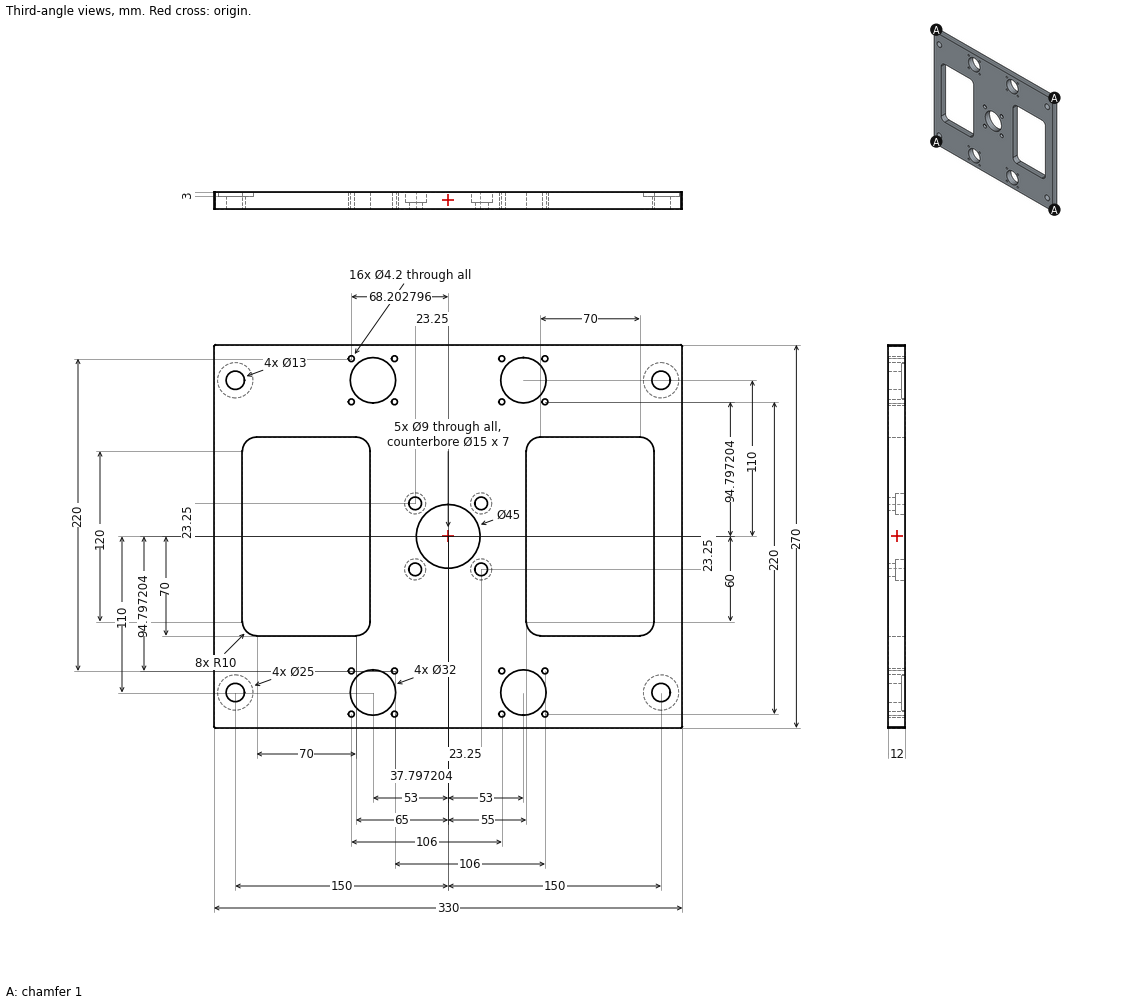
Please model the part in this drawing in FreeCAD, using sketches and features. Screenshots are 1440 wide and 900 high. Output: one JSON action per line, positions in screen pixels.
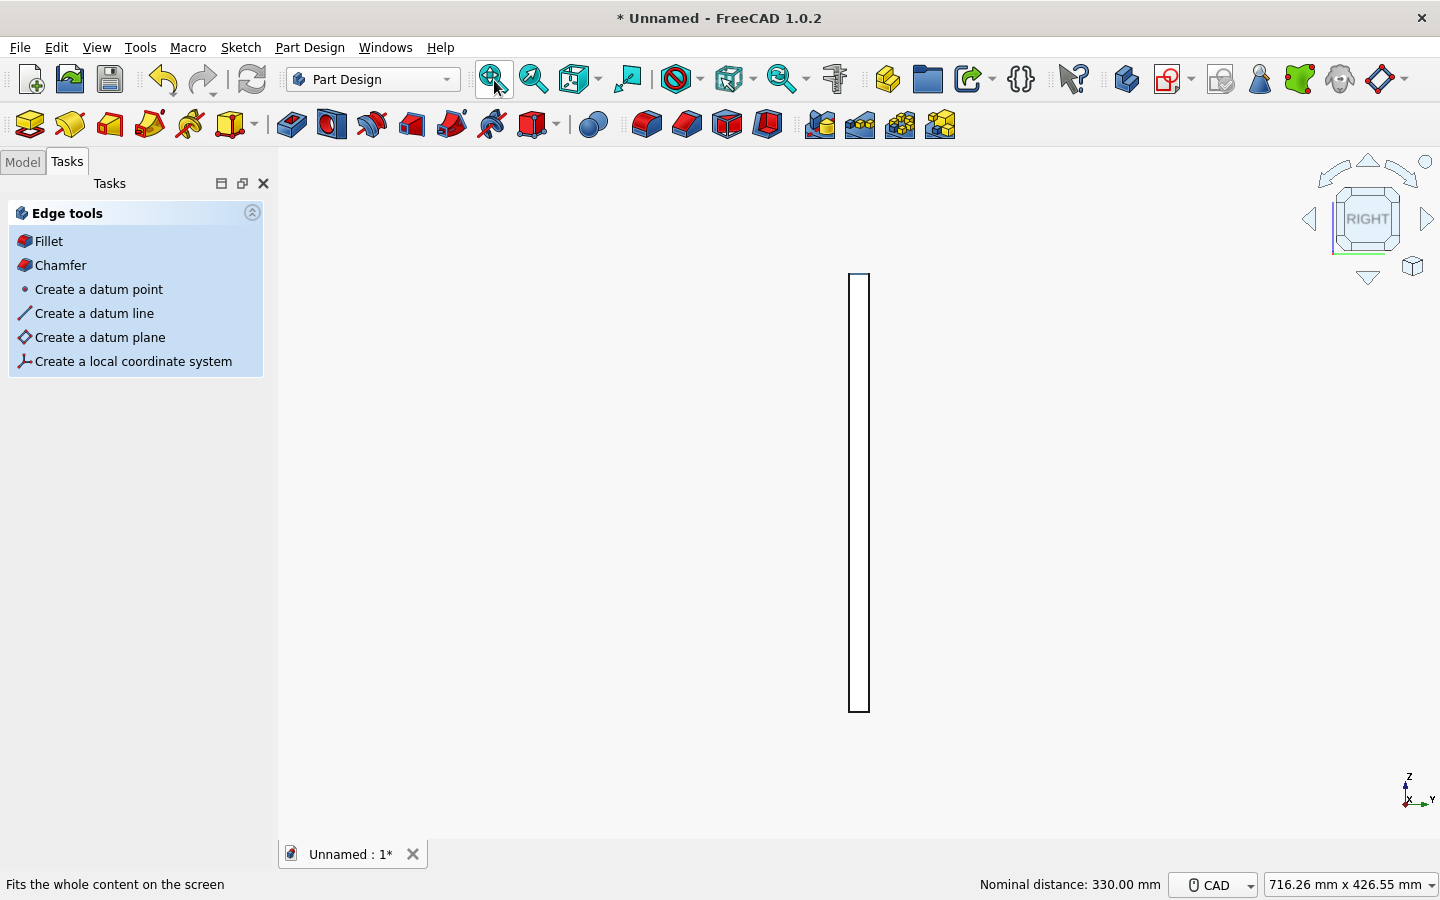
{"action": "left_click", "coordinate": [859, 711], "text": "ctrl"}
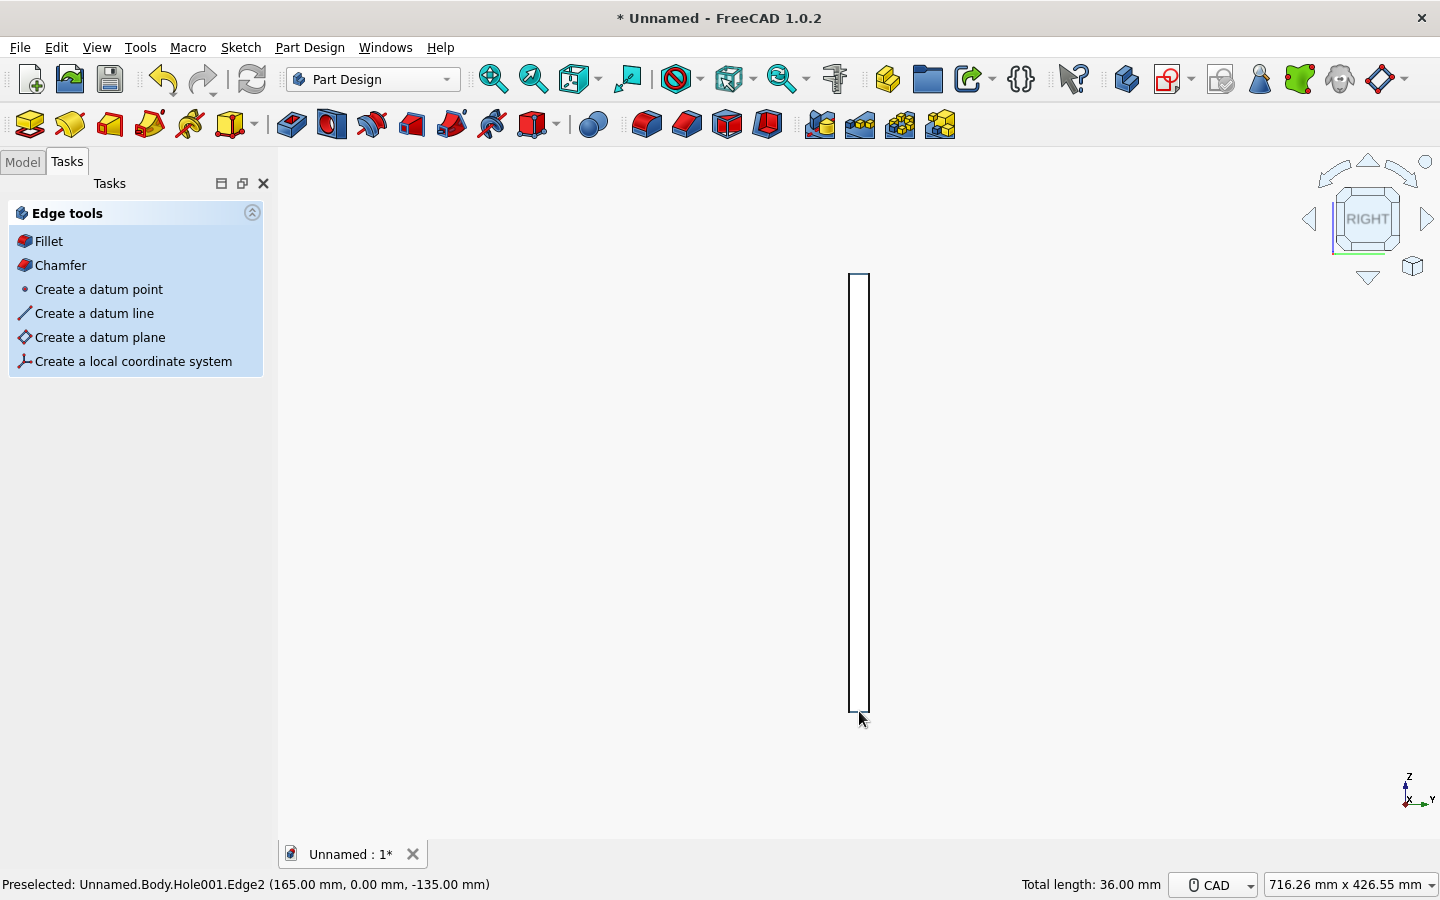
{"action": "scroll", "coordinate": [859, 711], "scroll_direction": "up", "scroll_amount": 4}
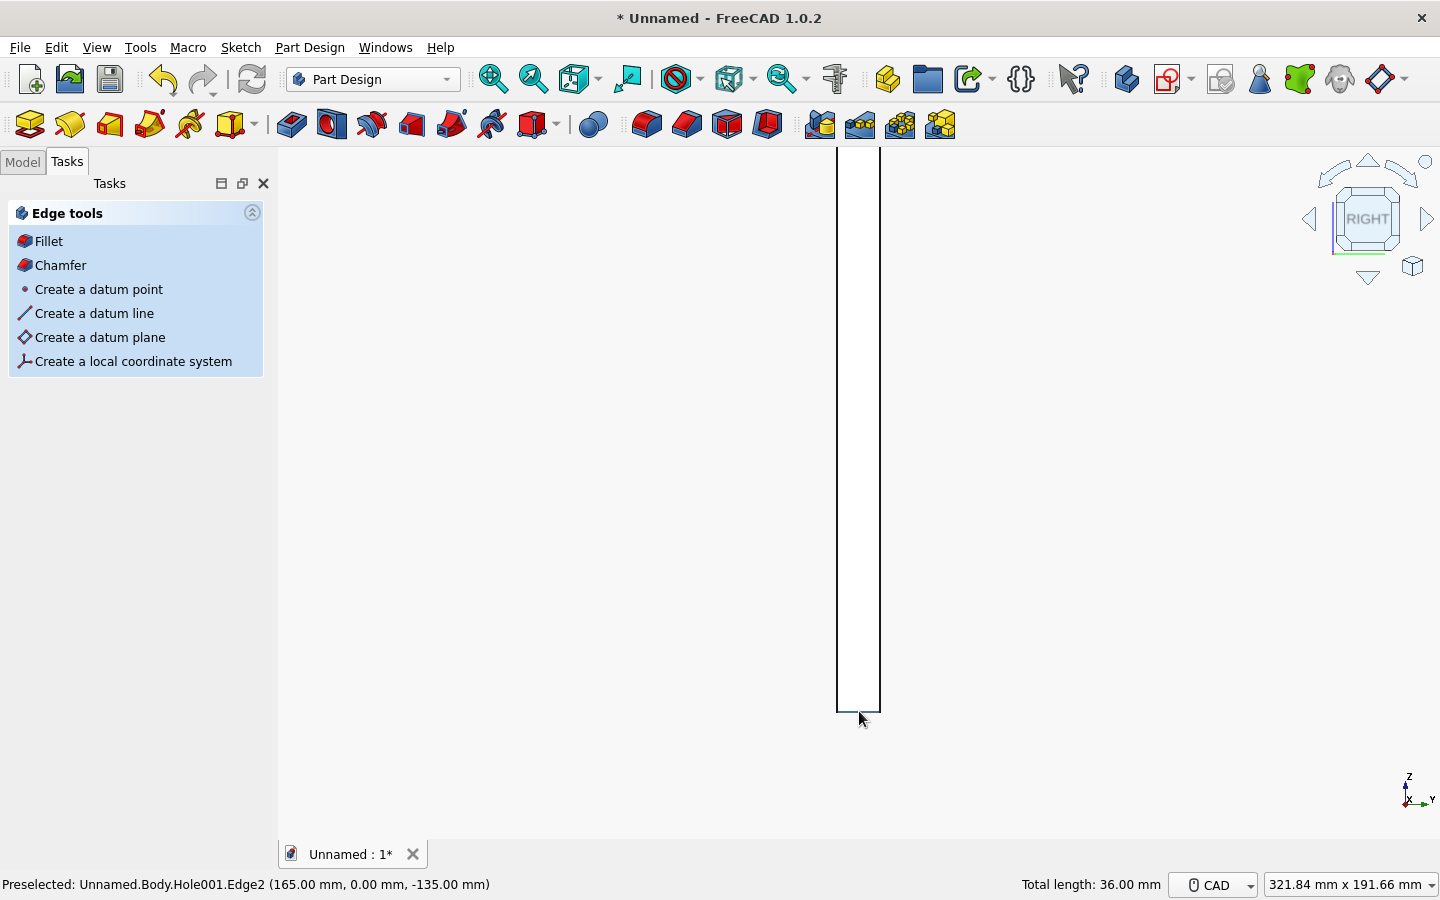
{"action": "left_click", "coordinate": [494, 80]}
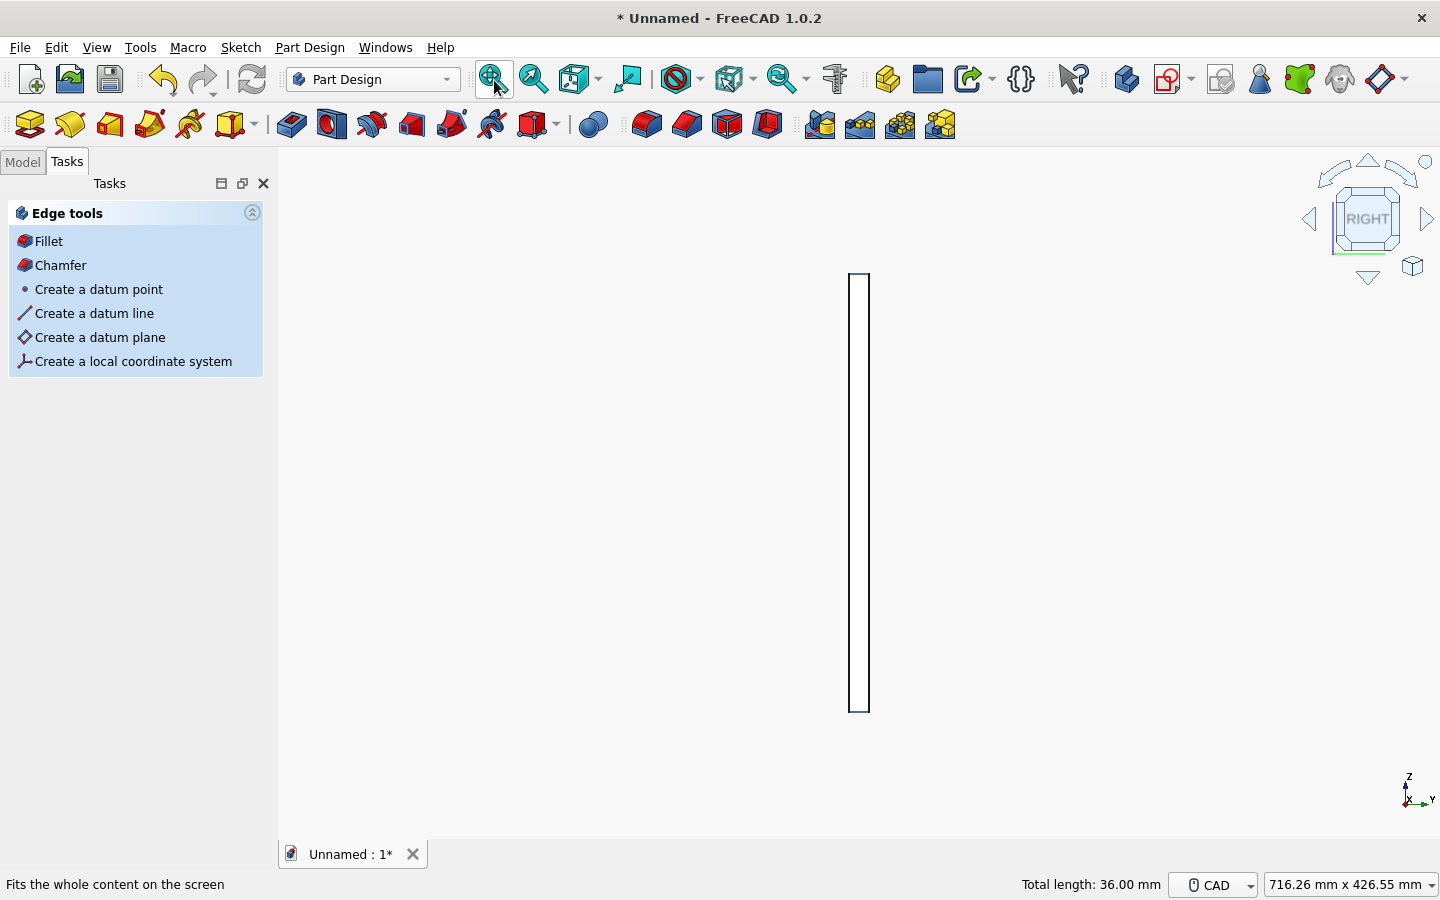
{"action": "key", "text": "5"}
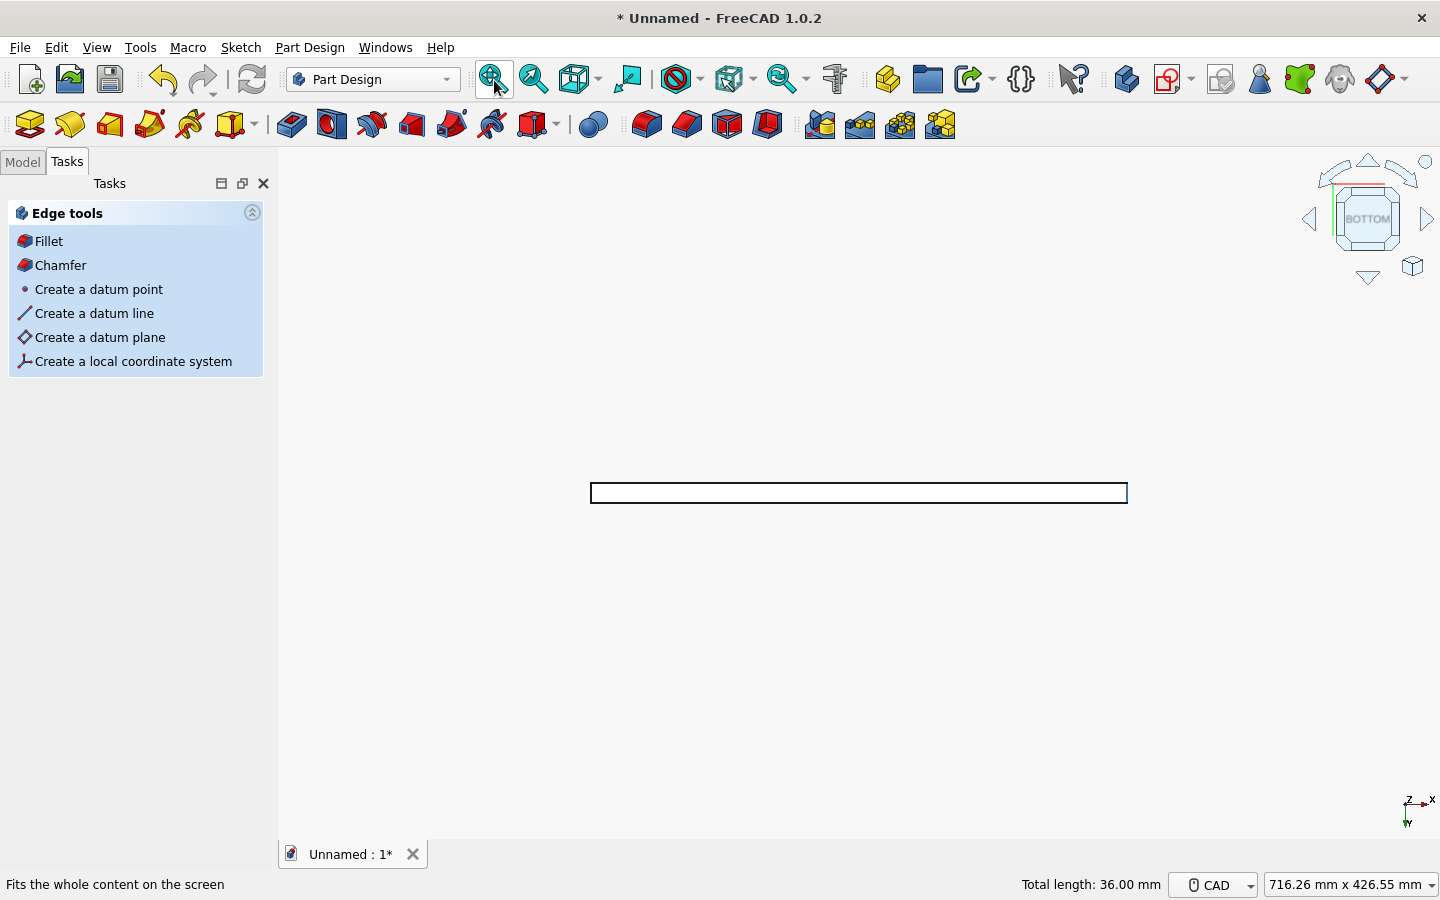
{"action": "left_click", "coordinate": [591, 492], "text": "ctrl"}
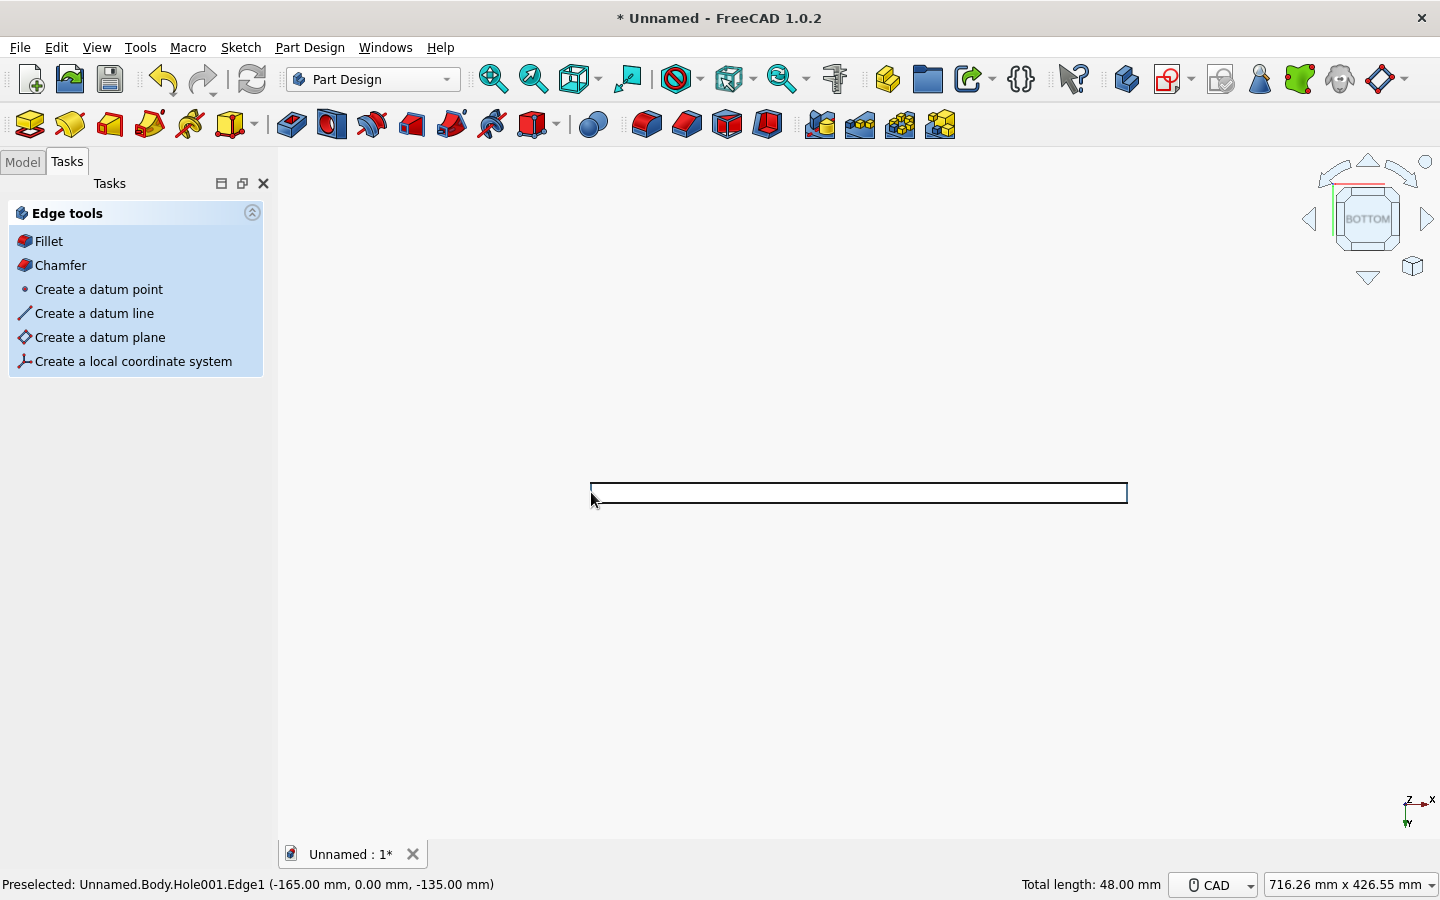
{"action": "left_click", "coordinate": [688, 124]}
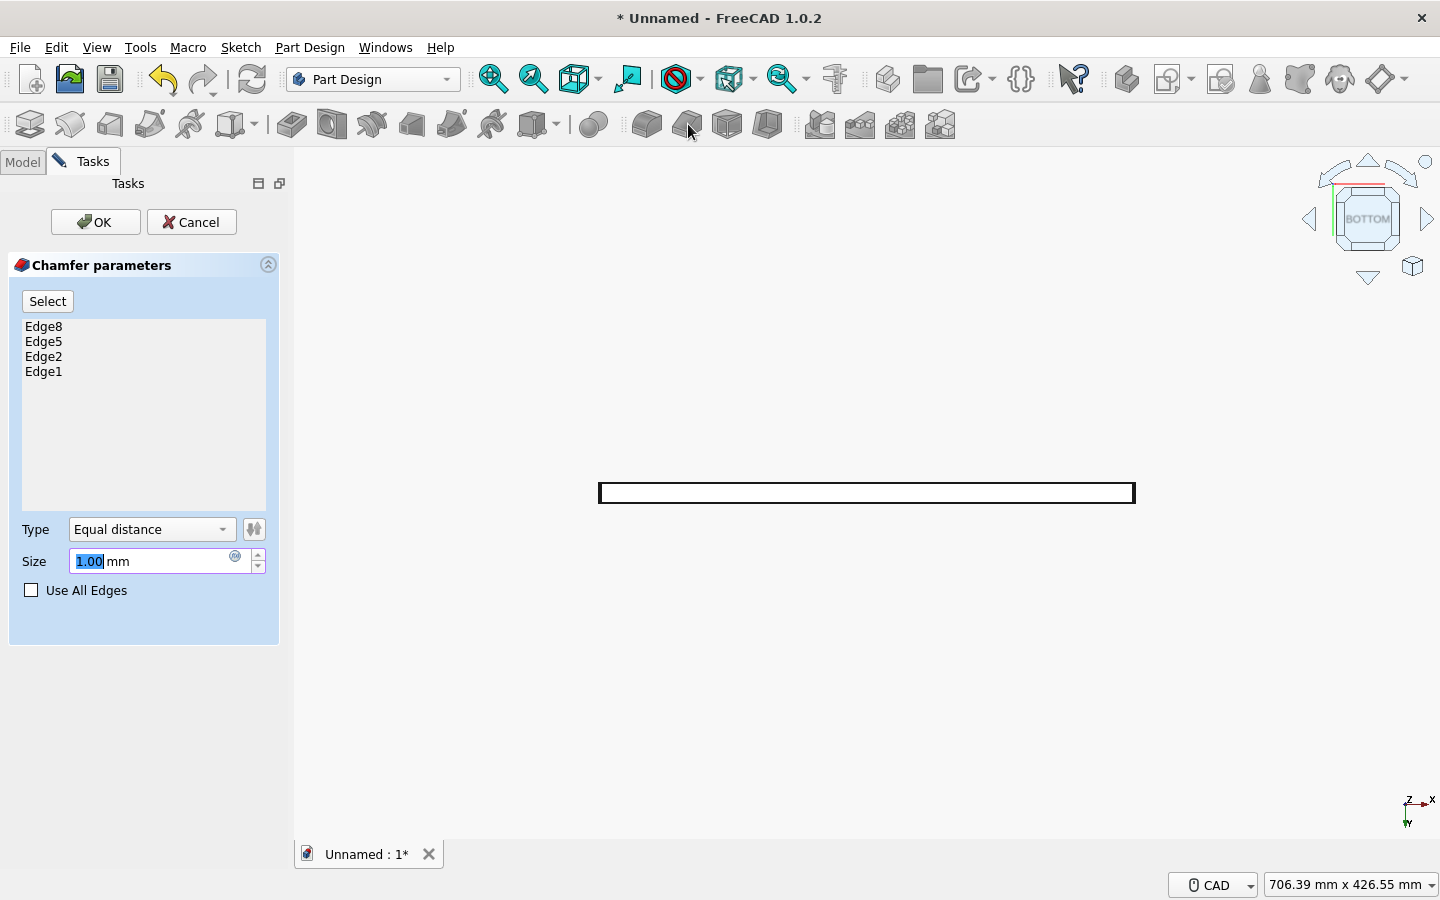
{"action": "type", "text": "1"}
{"action": "key", "text": "Tab"}